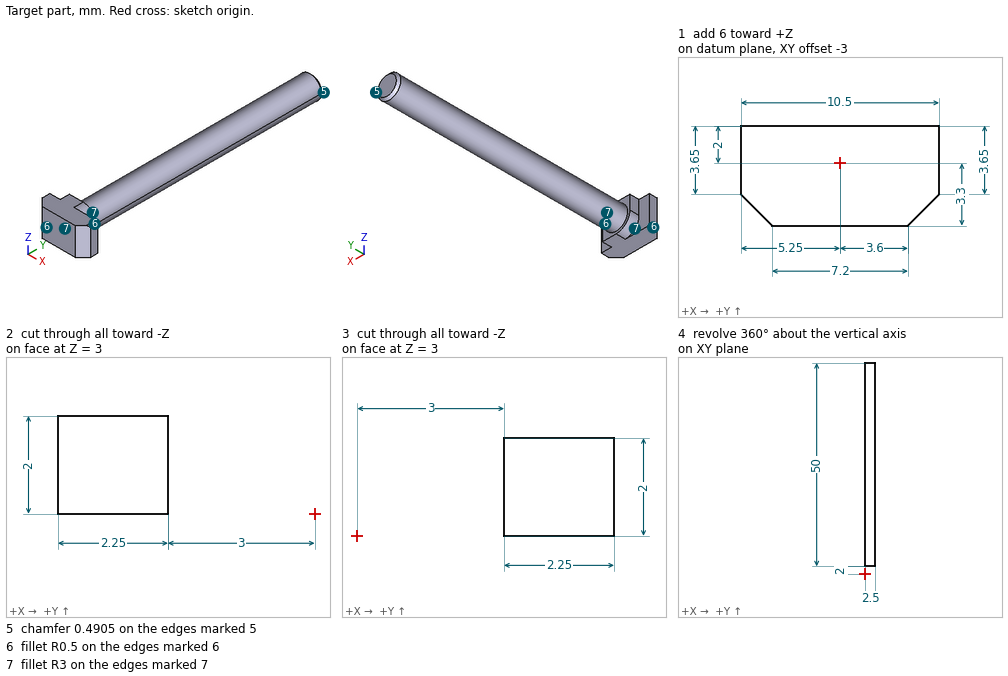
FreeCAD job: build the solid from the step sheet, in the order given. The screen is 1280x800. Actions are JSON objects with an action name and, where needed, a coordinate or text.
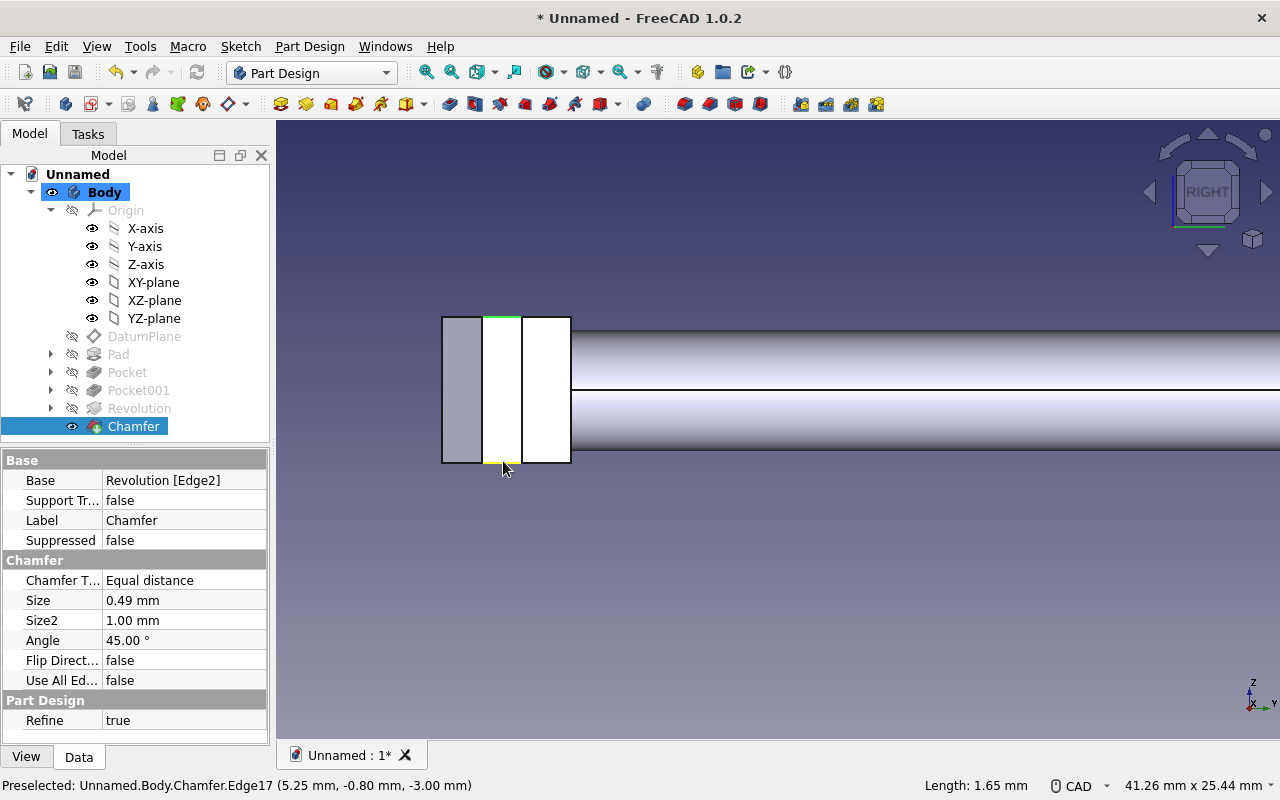
{"action": "key", "text": "v f"}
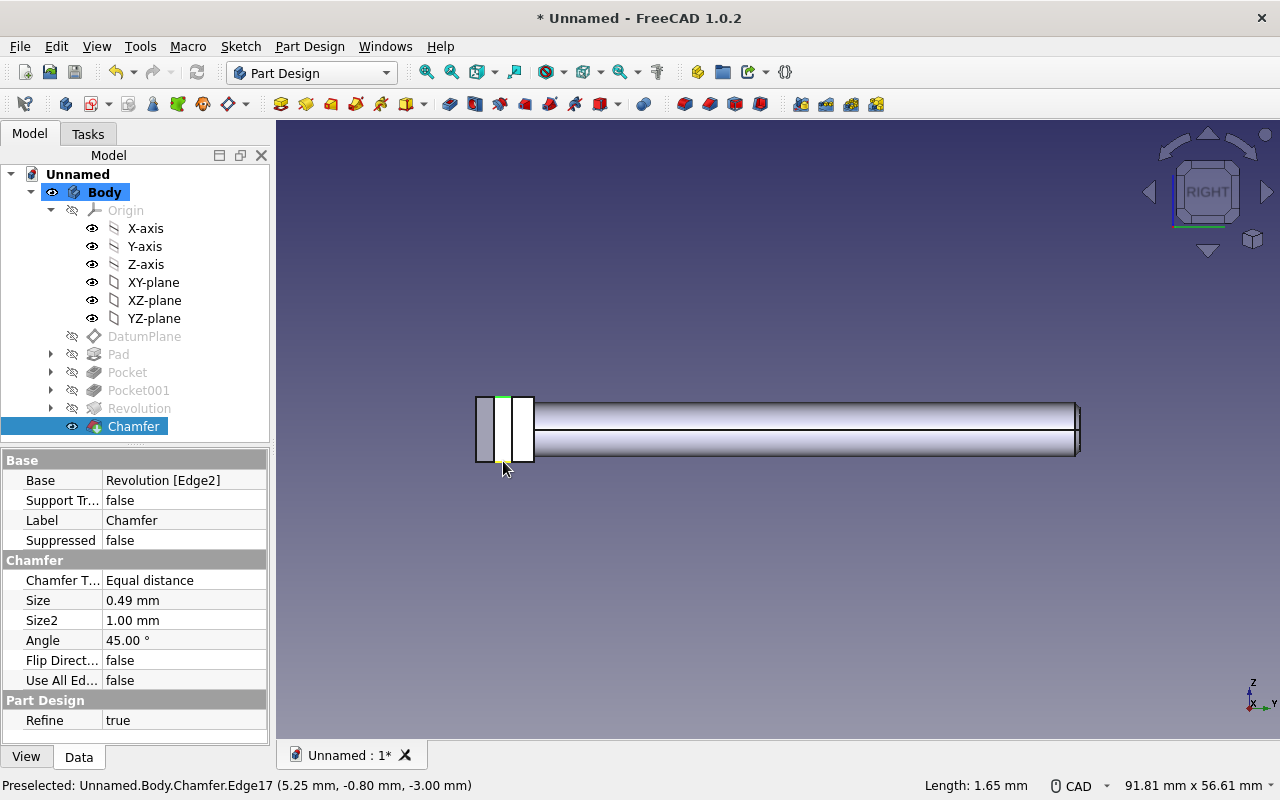
{"action": "key", "text": "0"}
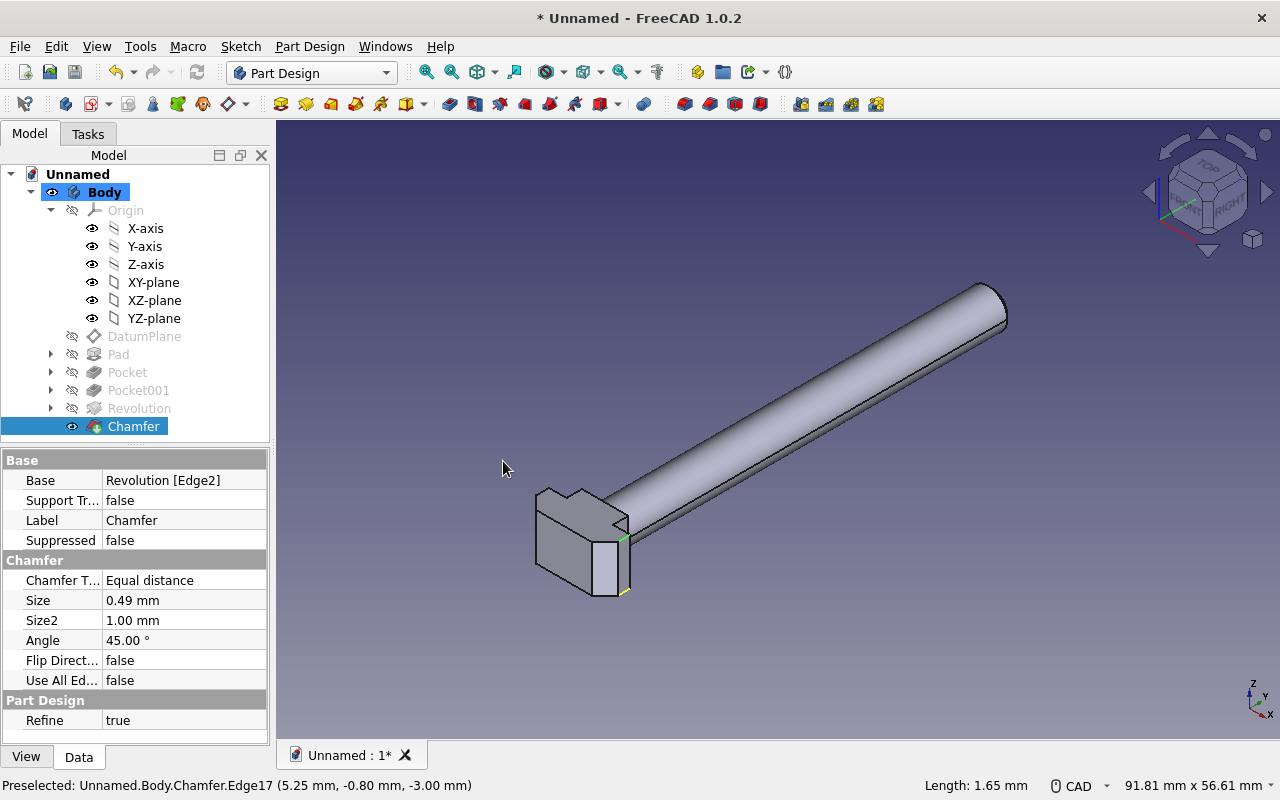
{"action": "scroll", "coordinate": [543, 544], "scroll_direction": "up", "scroll_amount": 4}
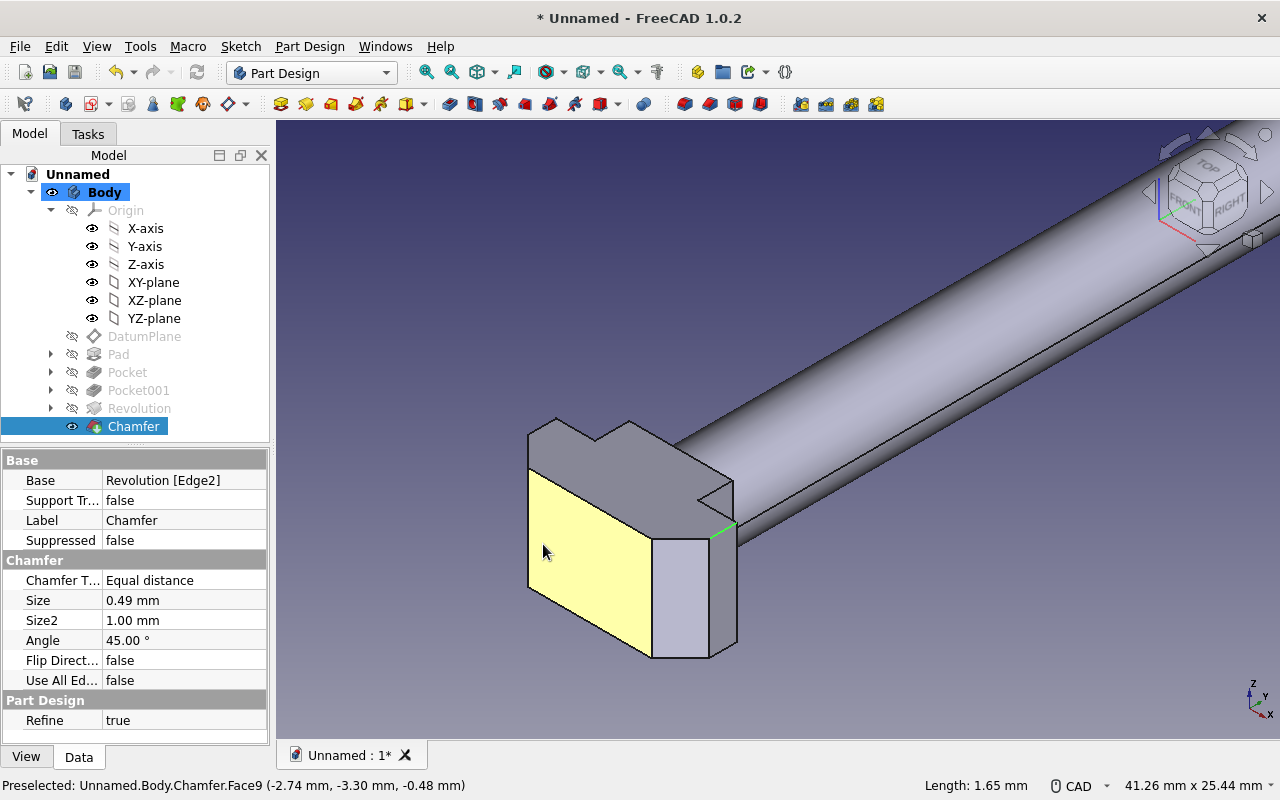
{"action": "key", "text": "v f"}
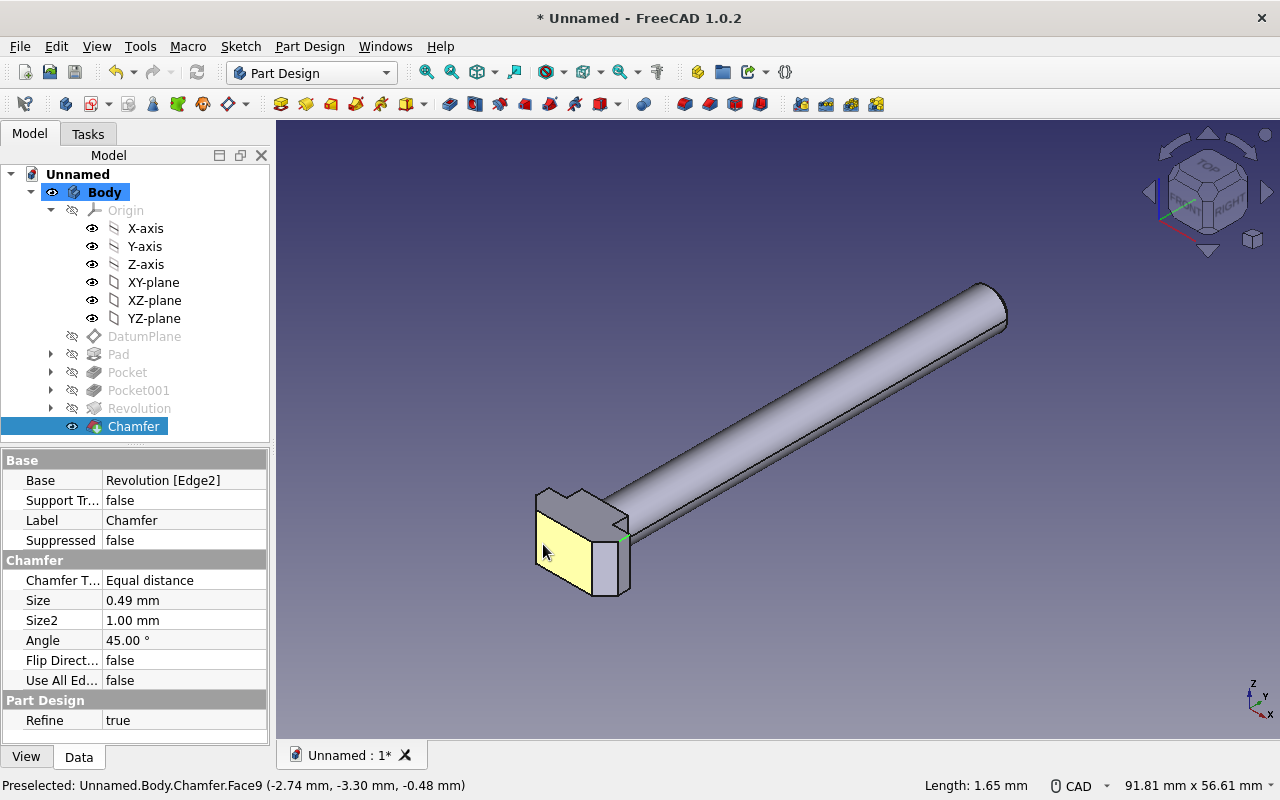
{"action": "key", "text": "2"}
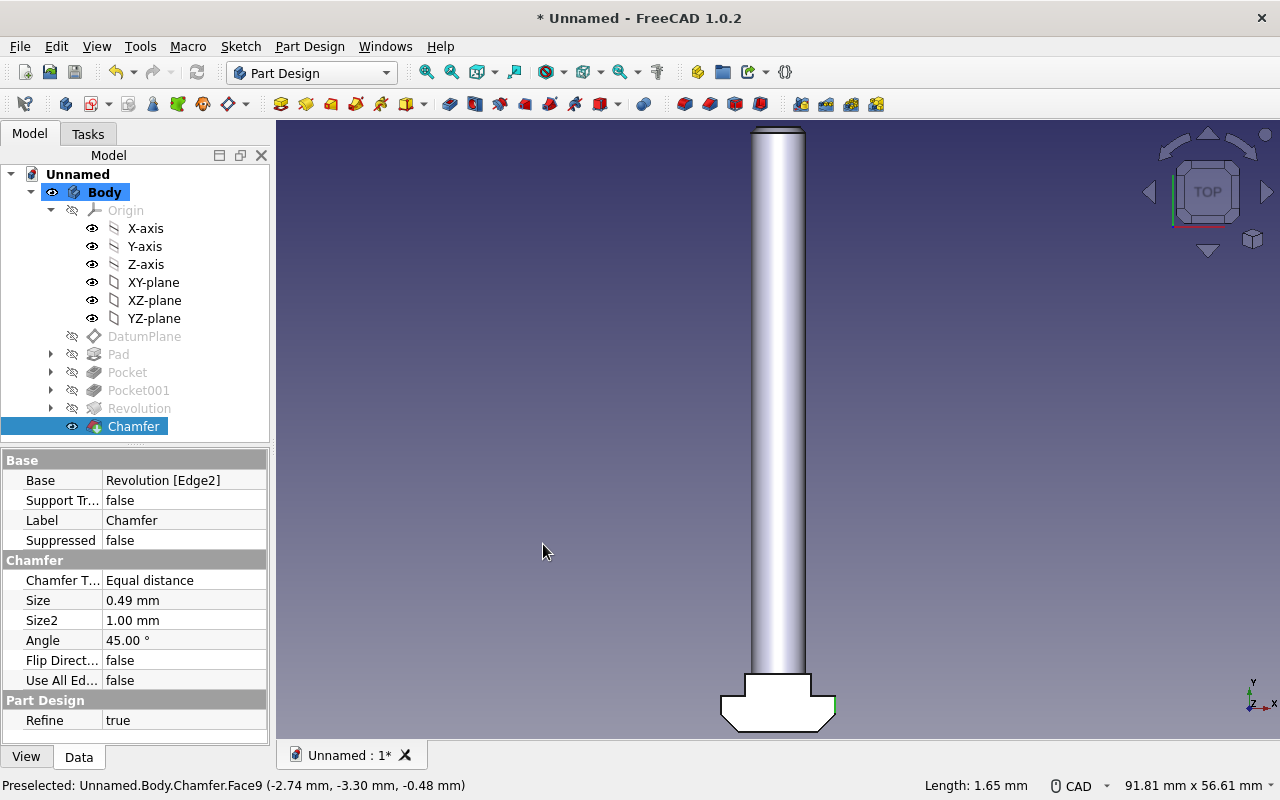
{"action": "scroll", "coordinate": [721, 704], "scroll_direction": "up", "scroll_amount": 4}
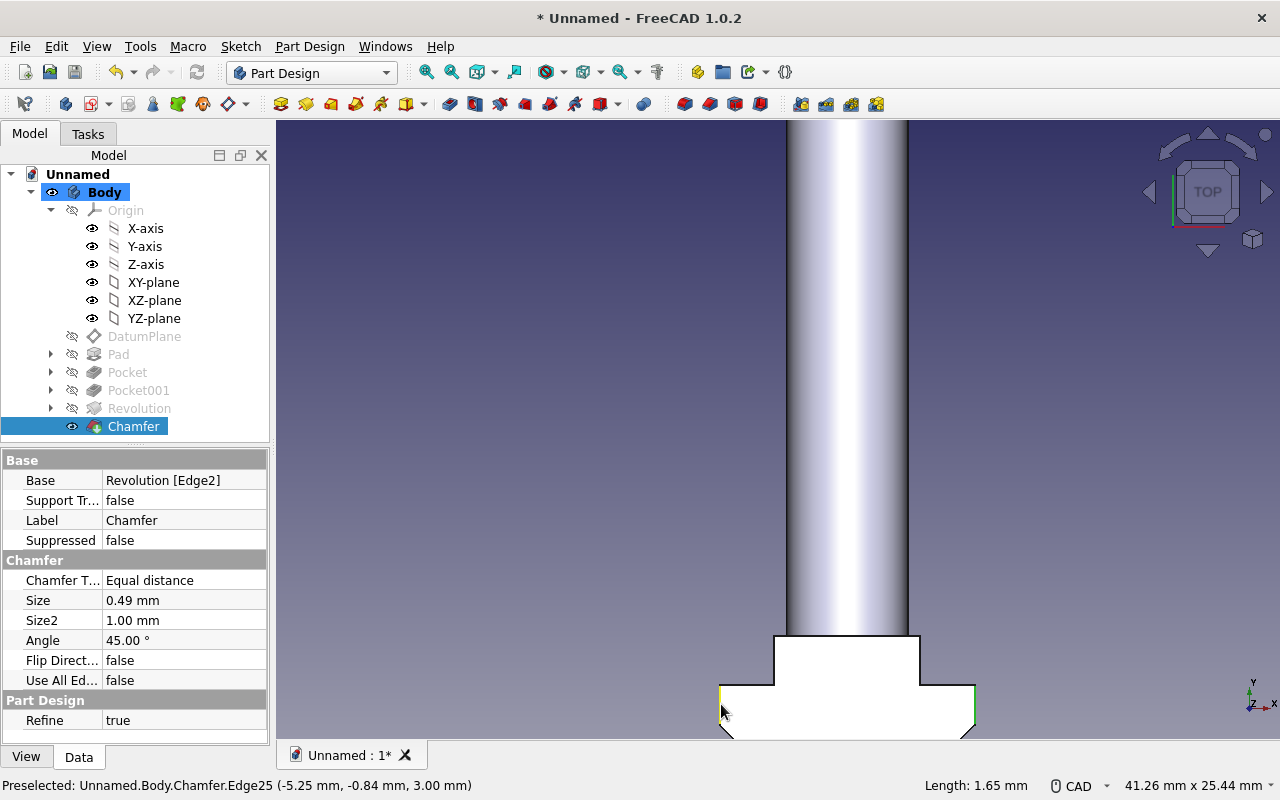
{"action": "key", "text": "v f"}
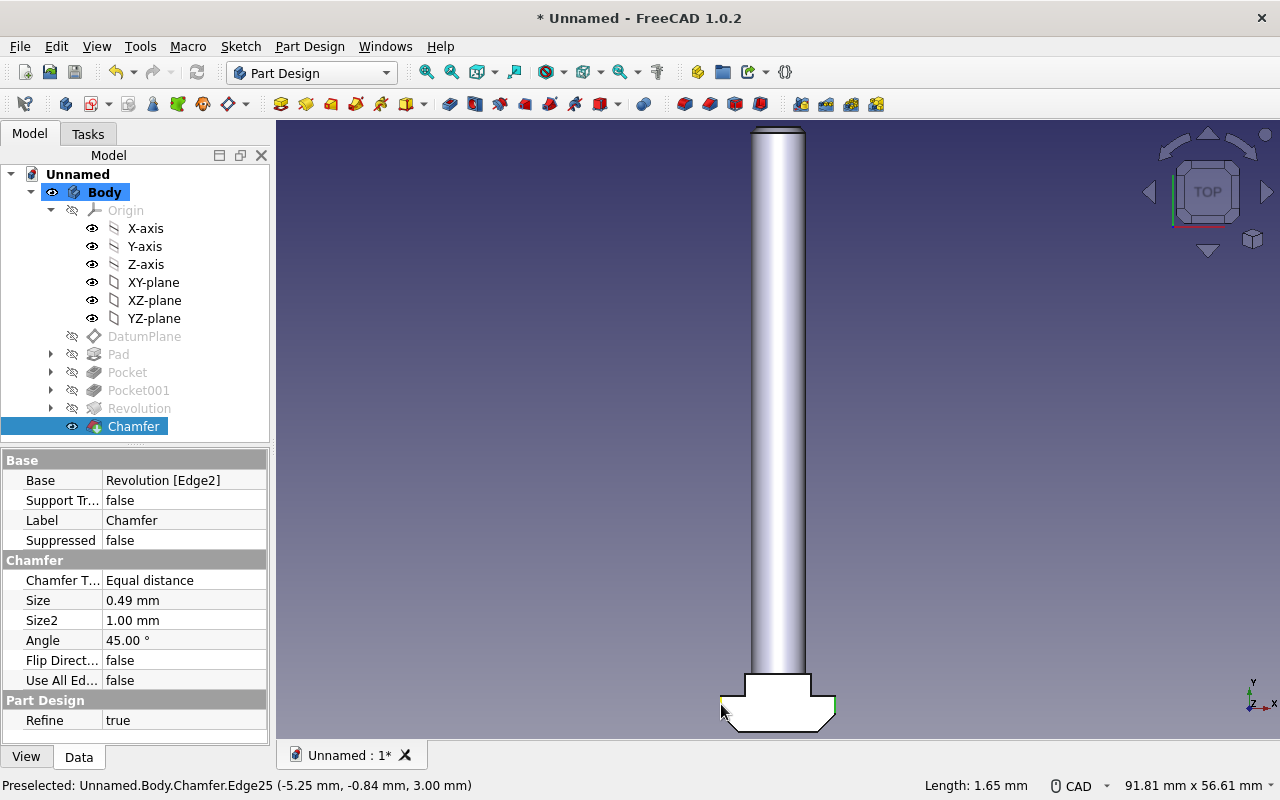
{"action": "key", "text": "1"}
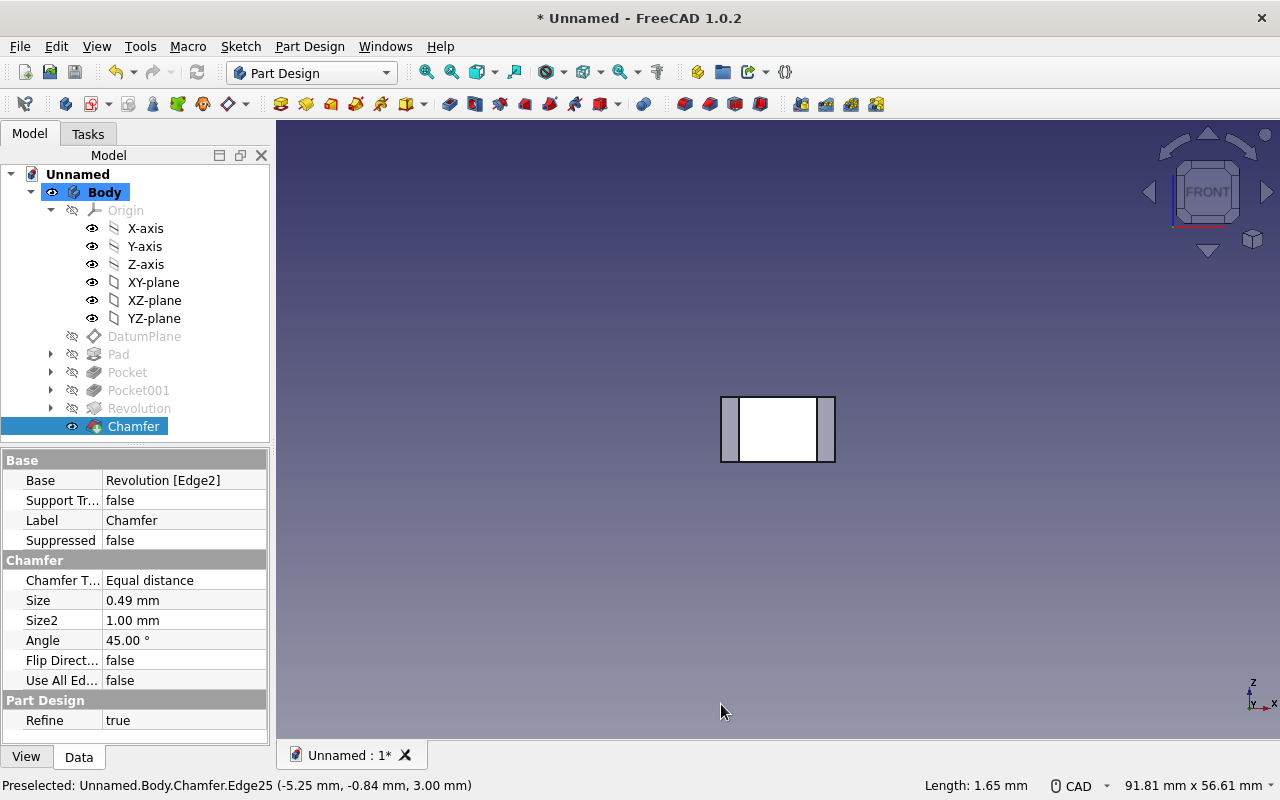
{"action": "left_click", "coordinate": [427, 72]}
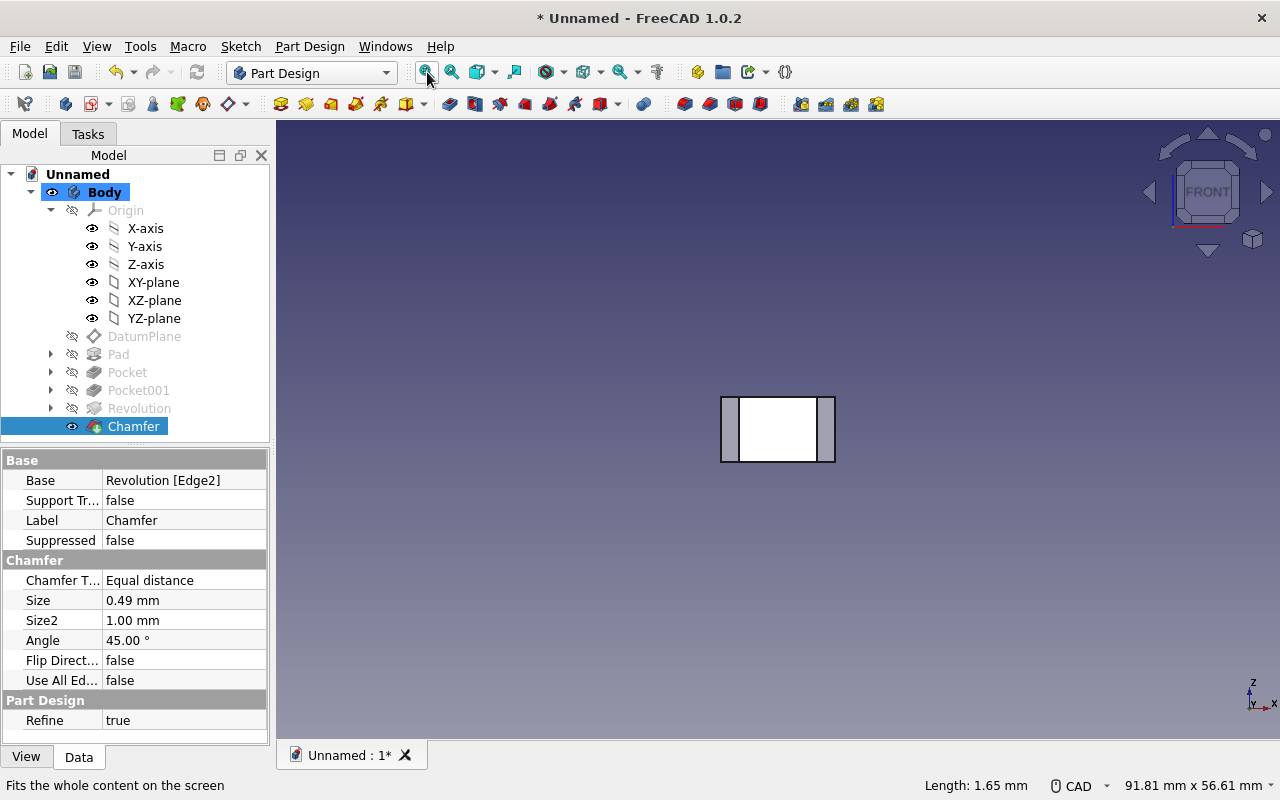
{"action": "scroll", "coordinate": [721, 461], "scroll_direction": "up", "scroll_amount": 4}